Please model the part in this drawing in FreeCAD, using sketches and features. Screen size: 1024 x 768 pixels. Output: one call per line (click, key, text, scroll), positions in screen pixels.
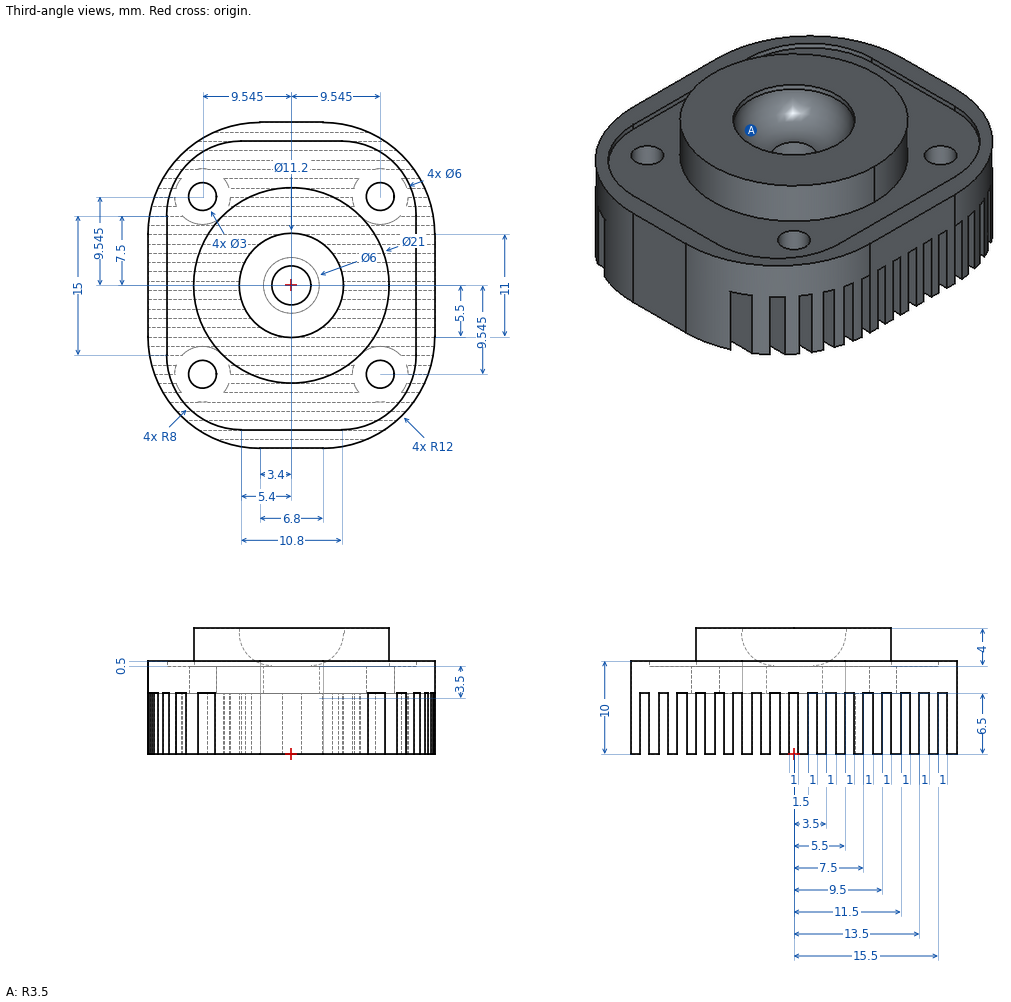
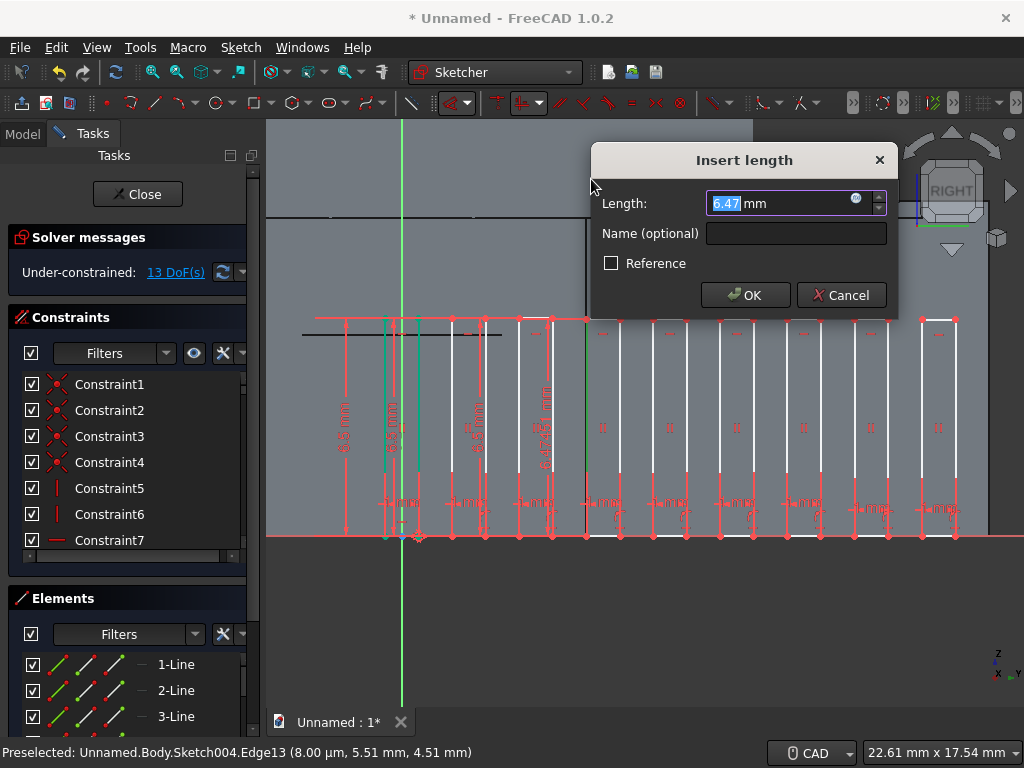
text(6.5)
key(Return)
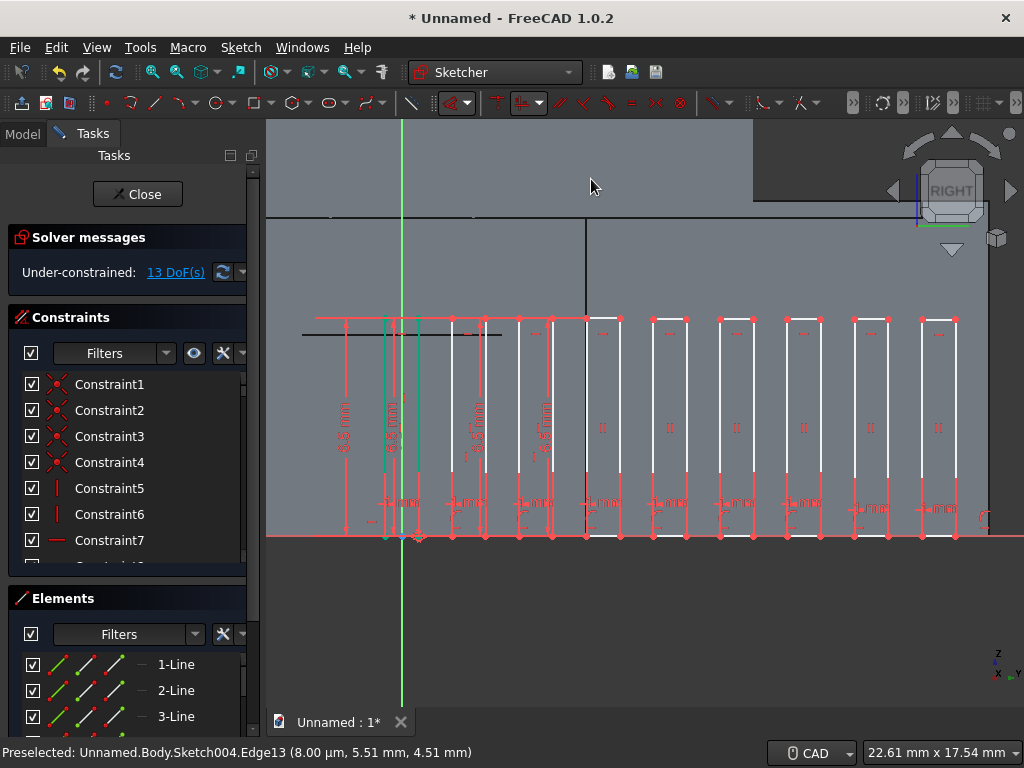
click(653, 384)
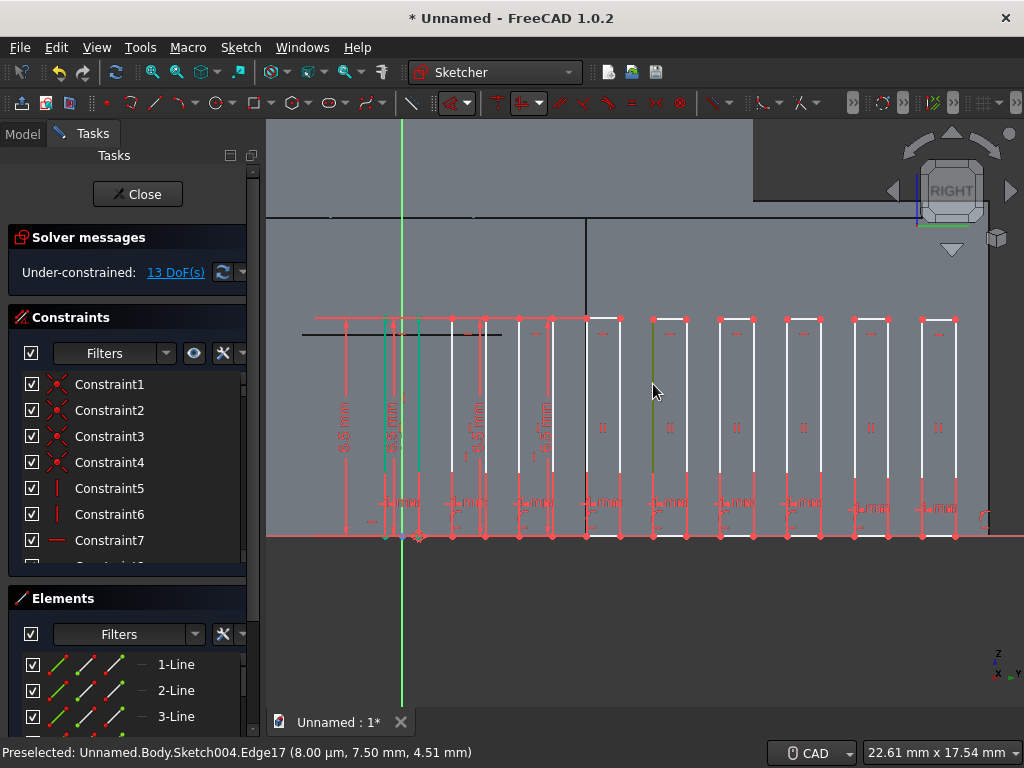
click(470, 104)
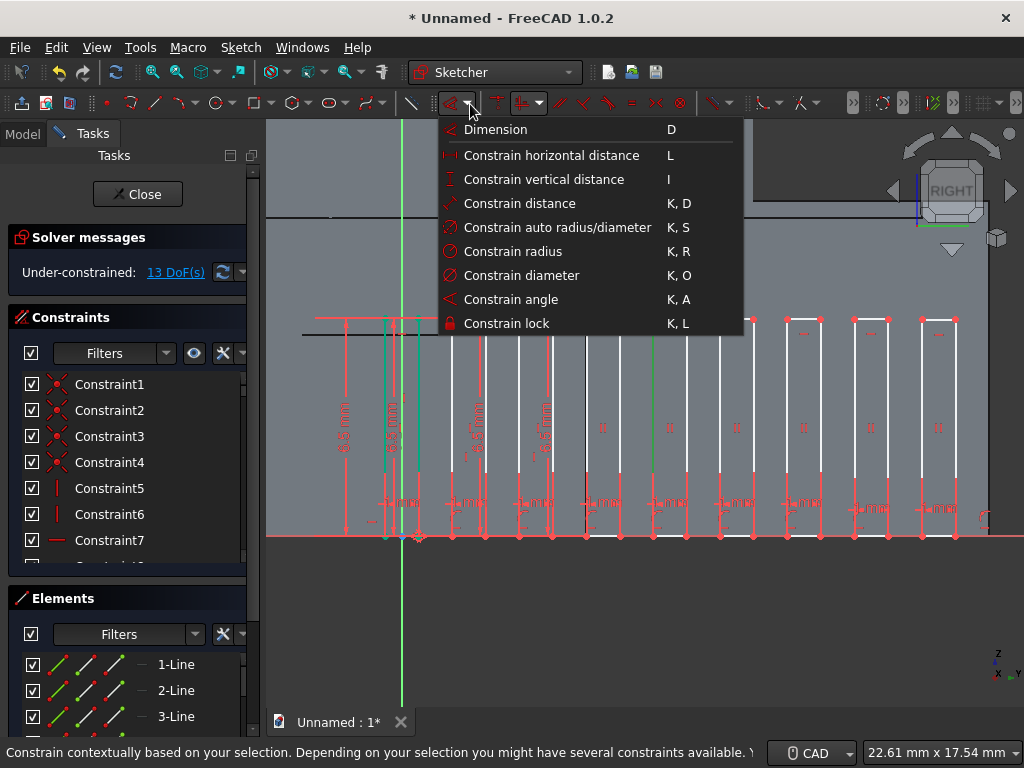
click(591, 179)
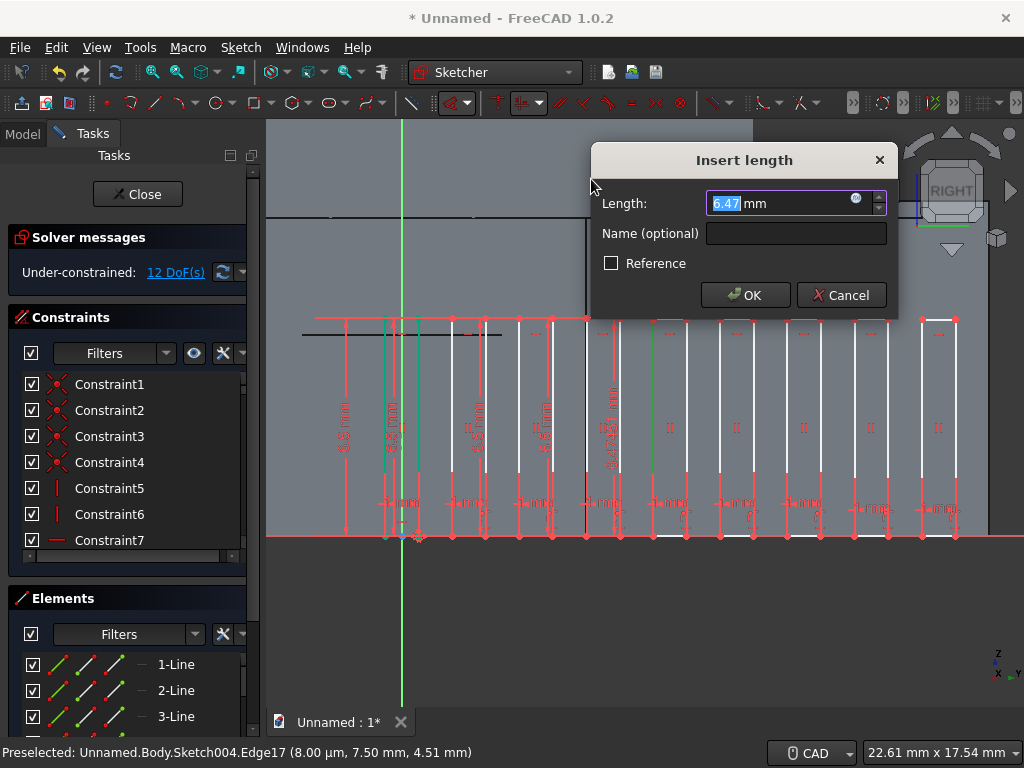
text(6.5)
key(Return)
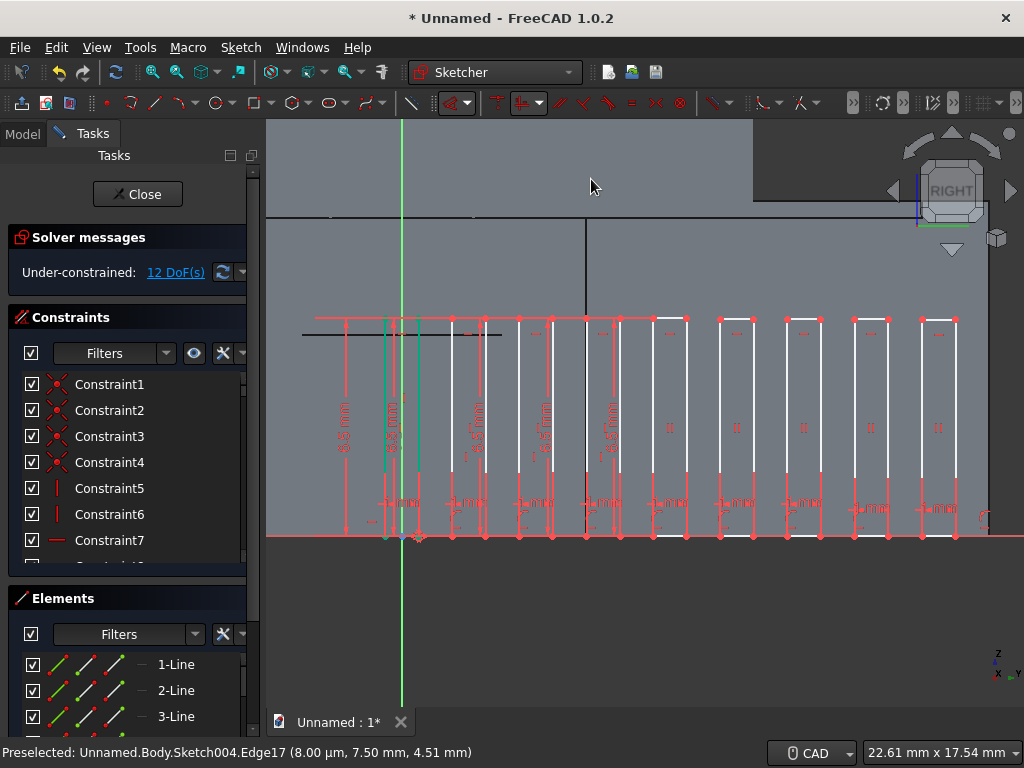
click(720, 384)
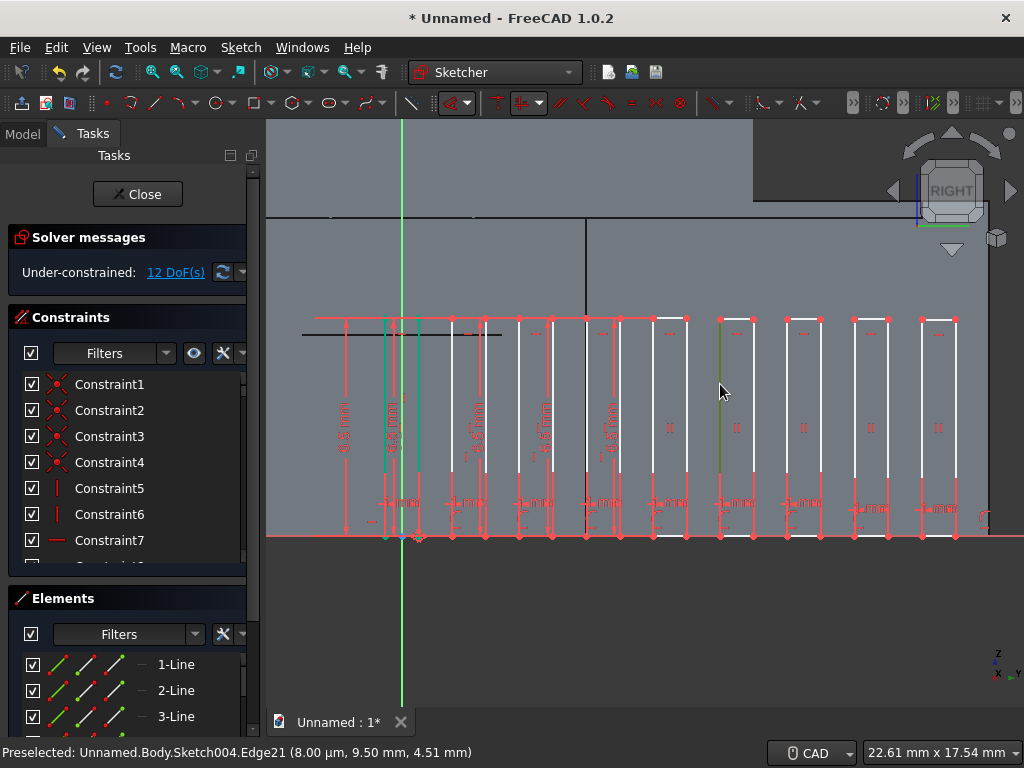
click(470, 104)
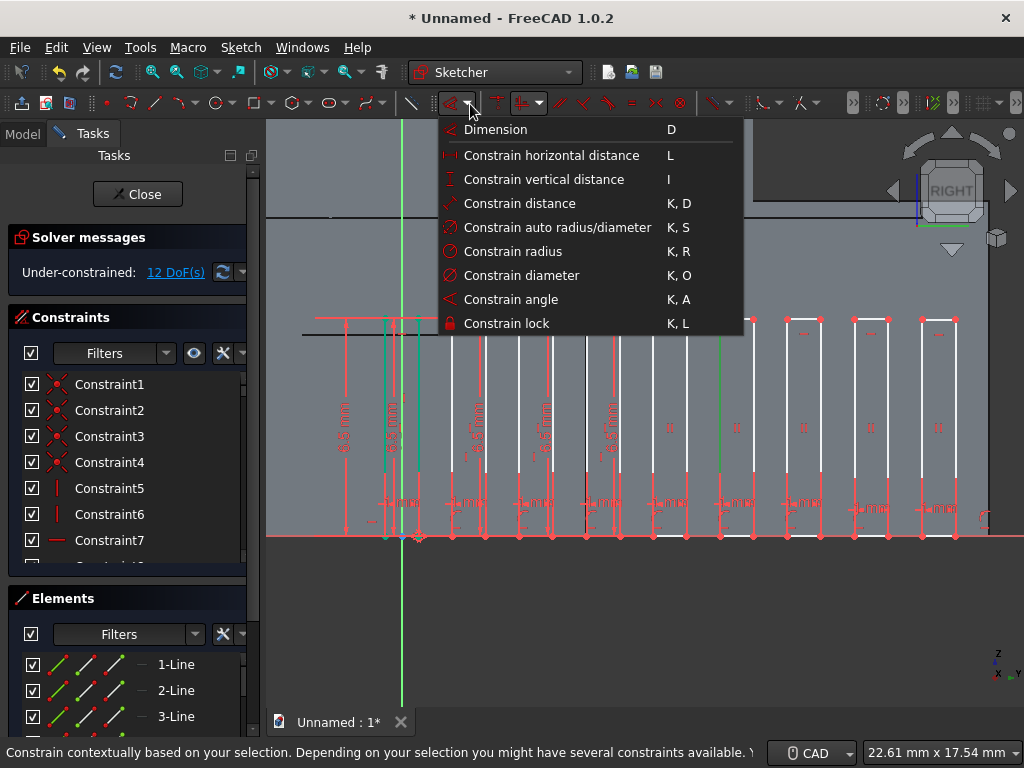
click(591, 179)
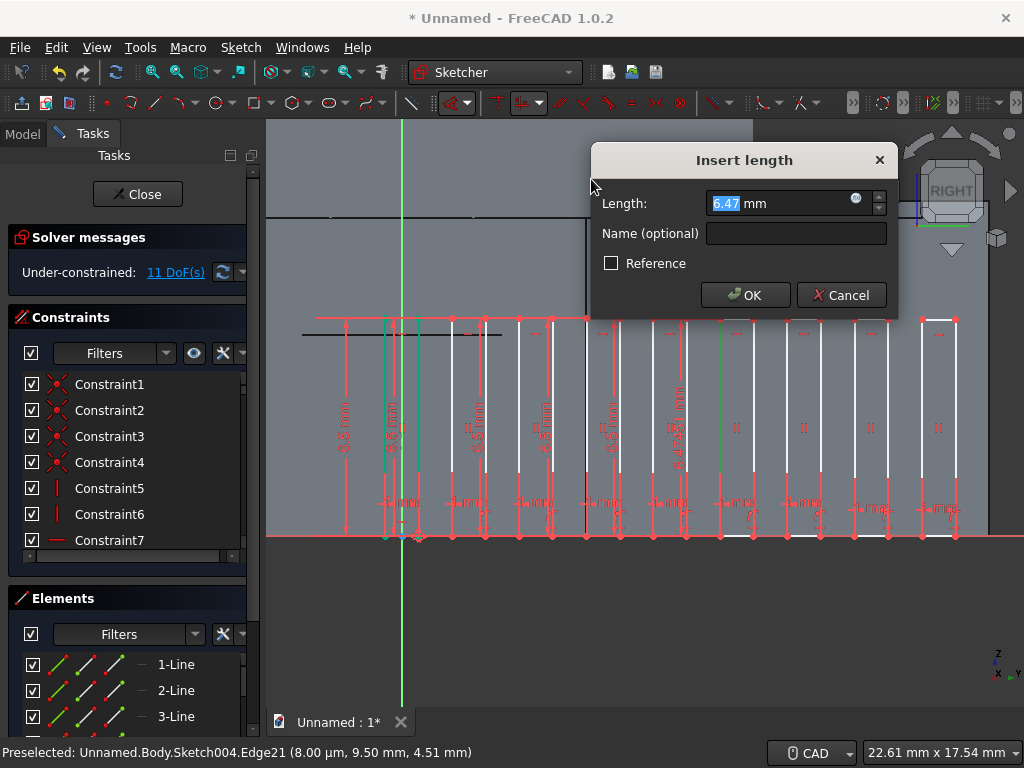
text(6.5)
key(Return)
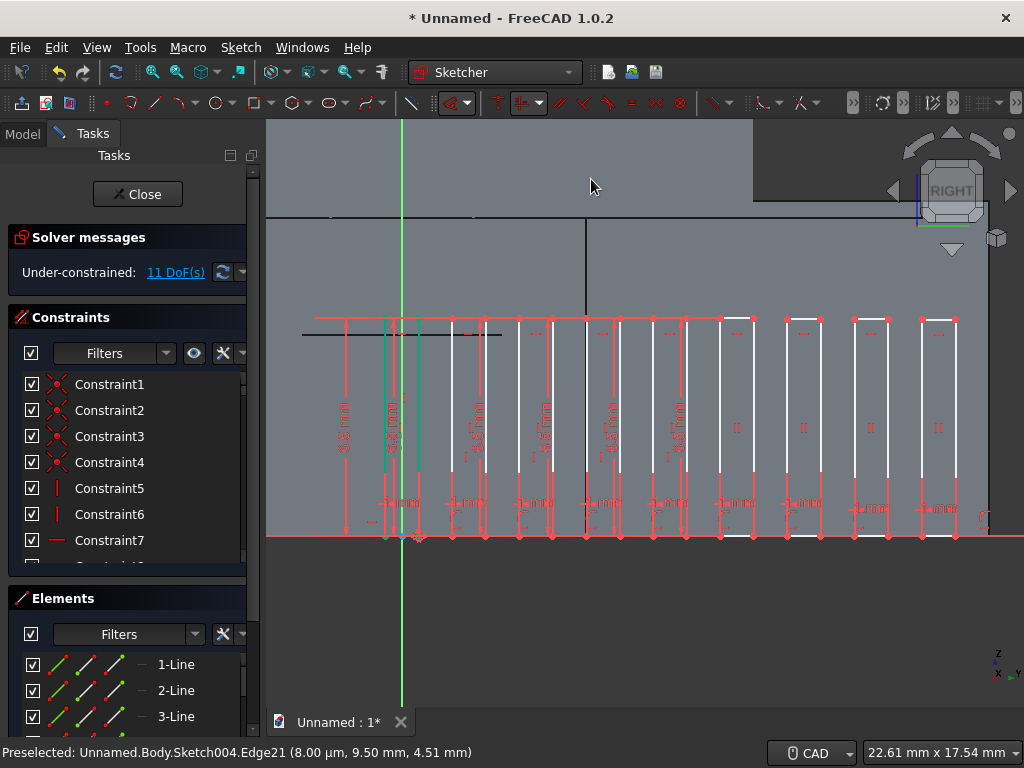
click(787, 384)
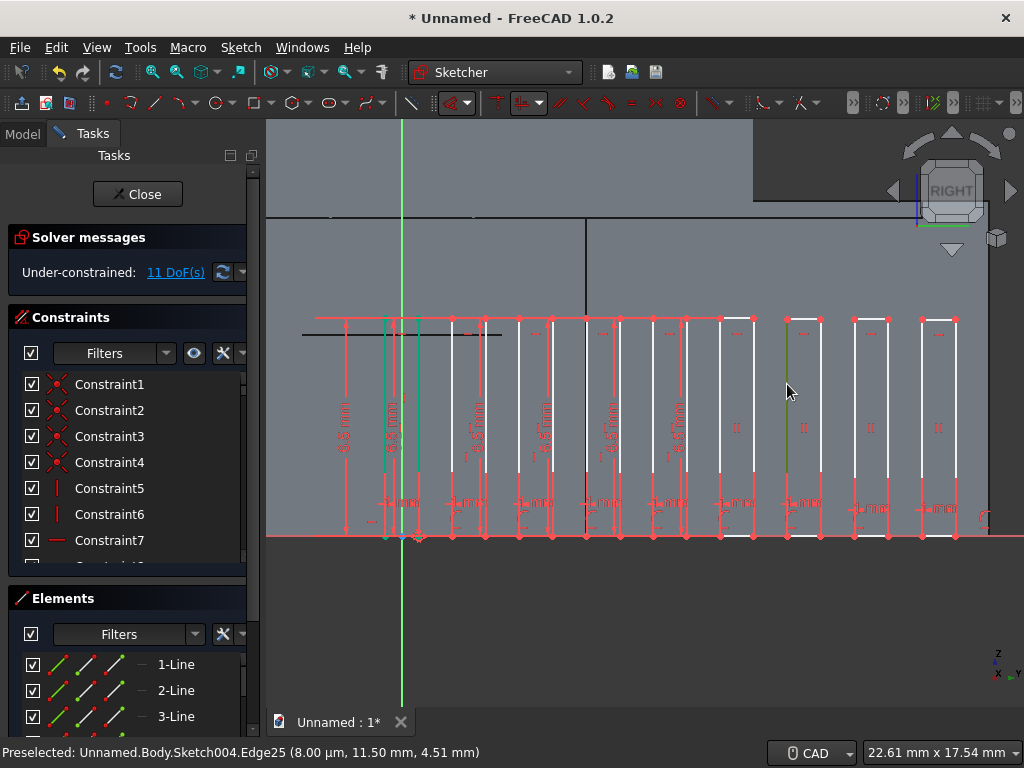
click(470, 104)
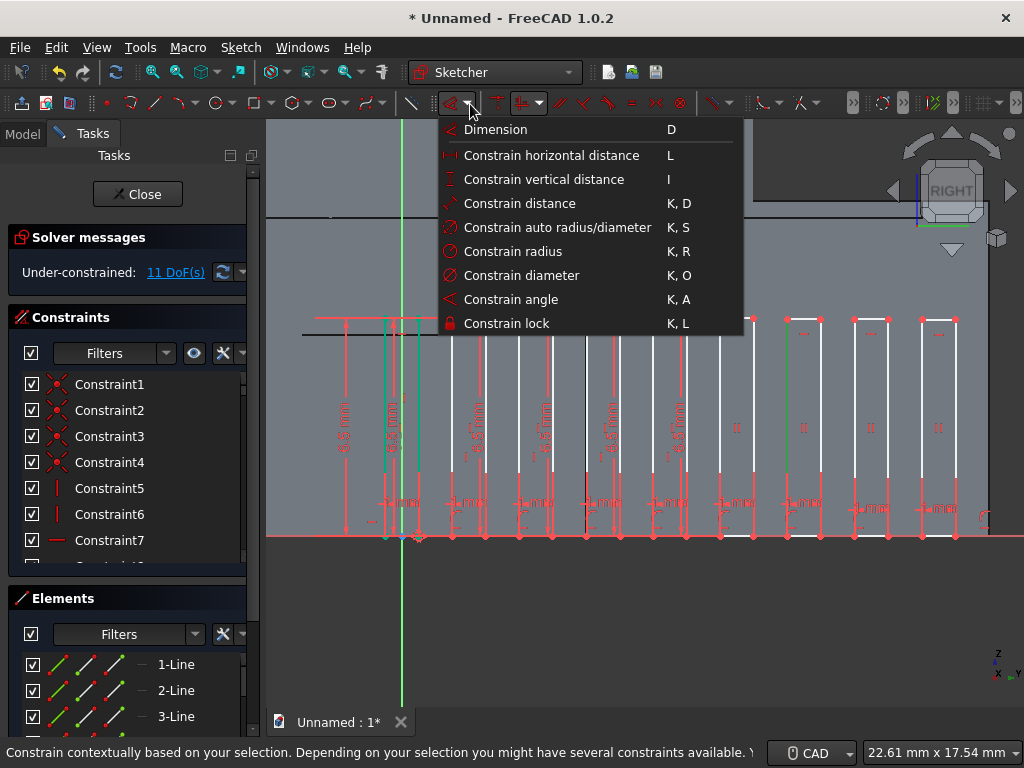
click(591, 179)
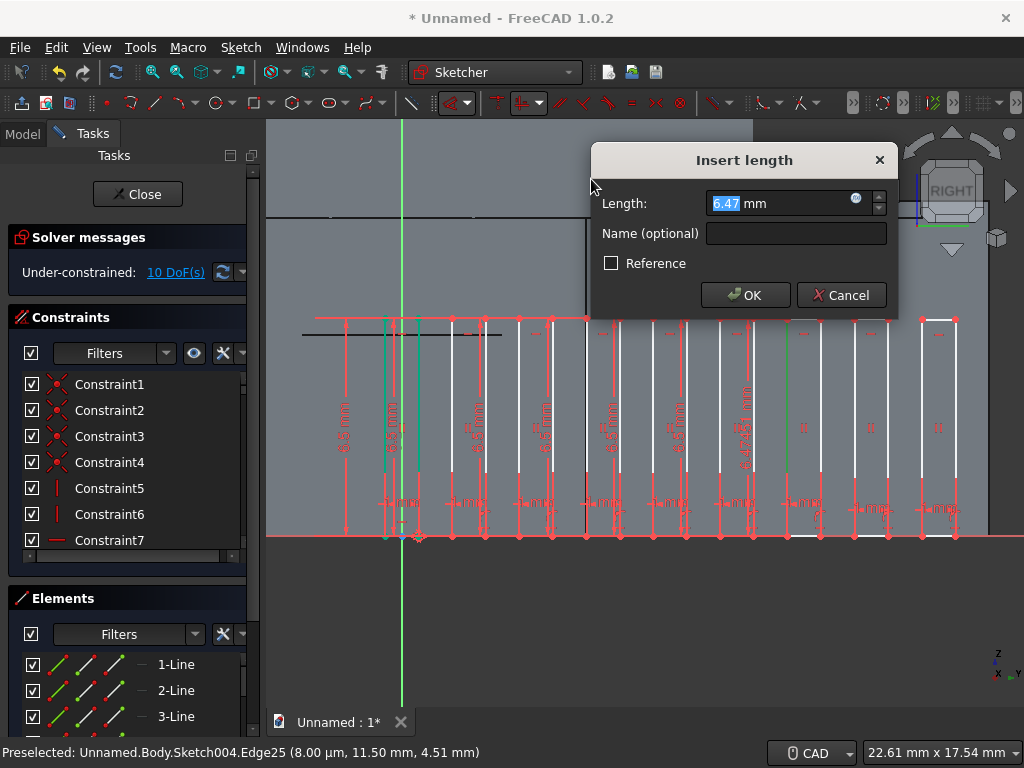
text(6.5)
key(Return)